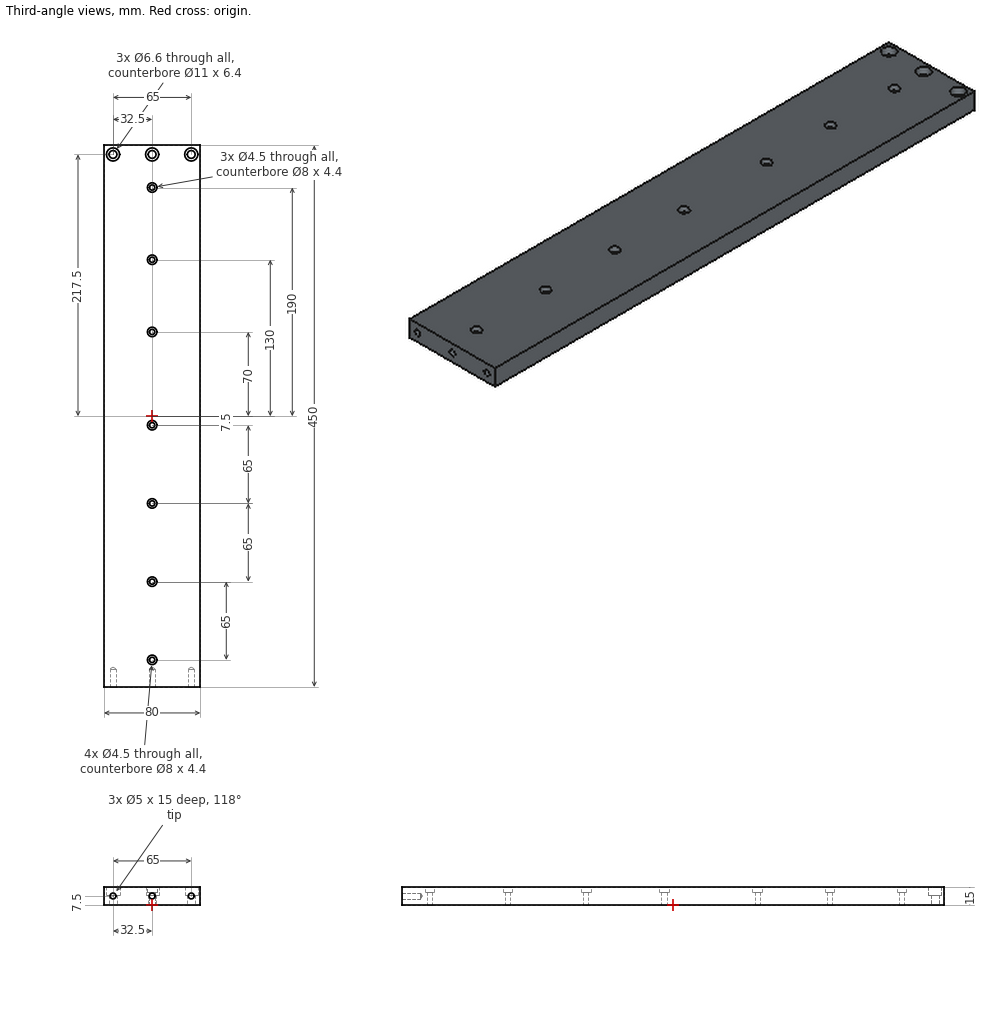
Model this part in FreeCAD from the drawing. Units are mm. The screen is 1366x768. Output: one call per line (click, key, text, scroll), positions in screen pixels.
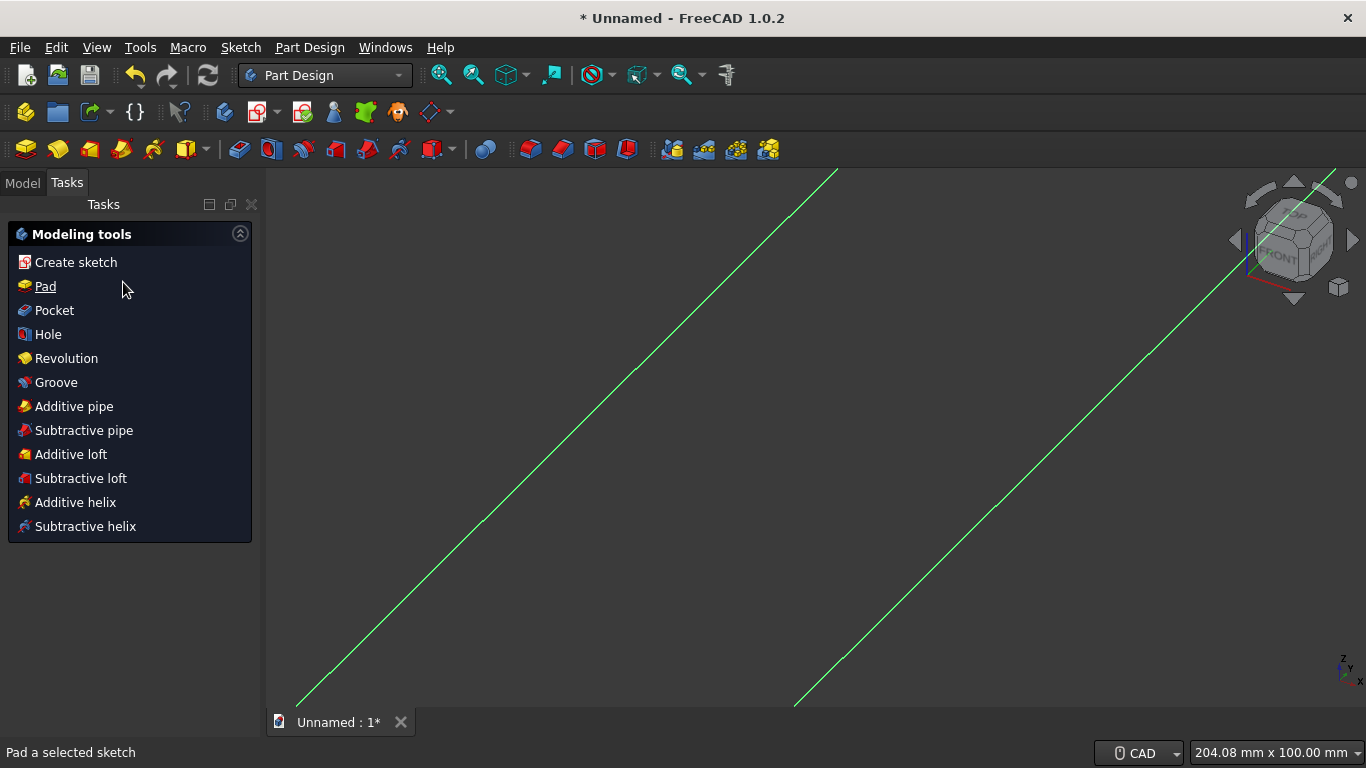
click(26, 150)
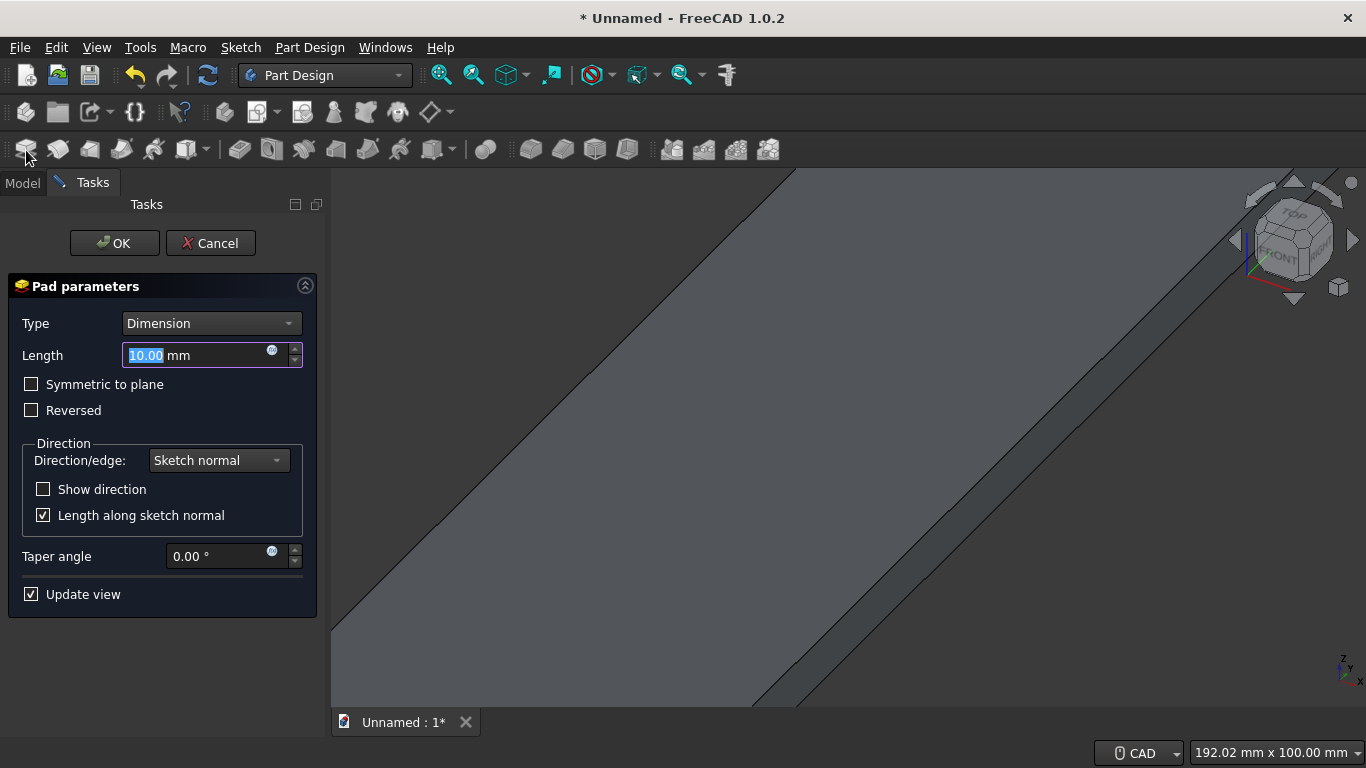
text(15)
key(Tab)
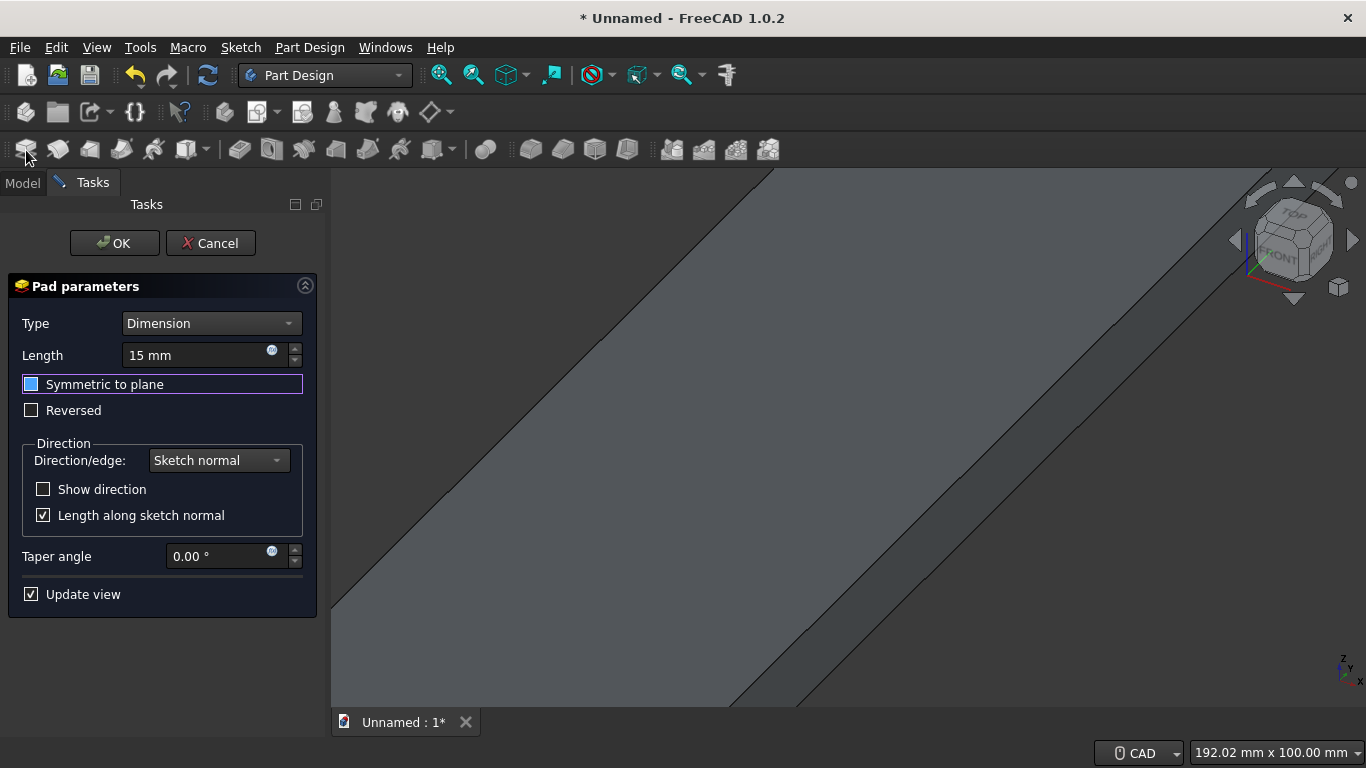
click(115, 243)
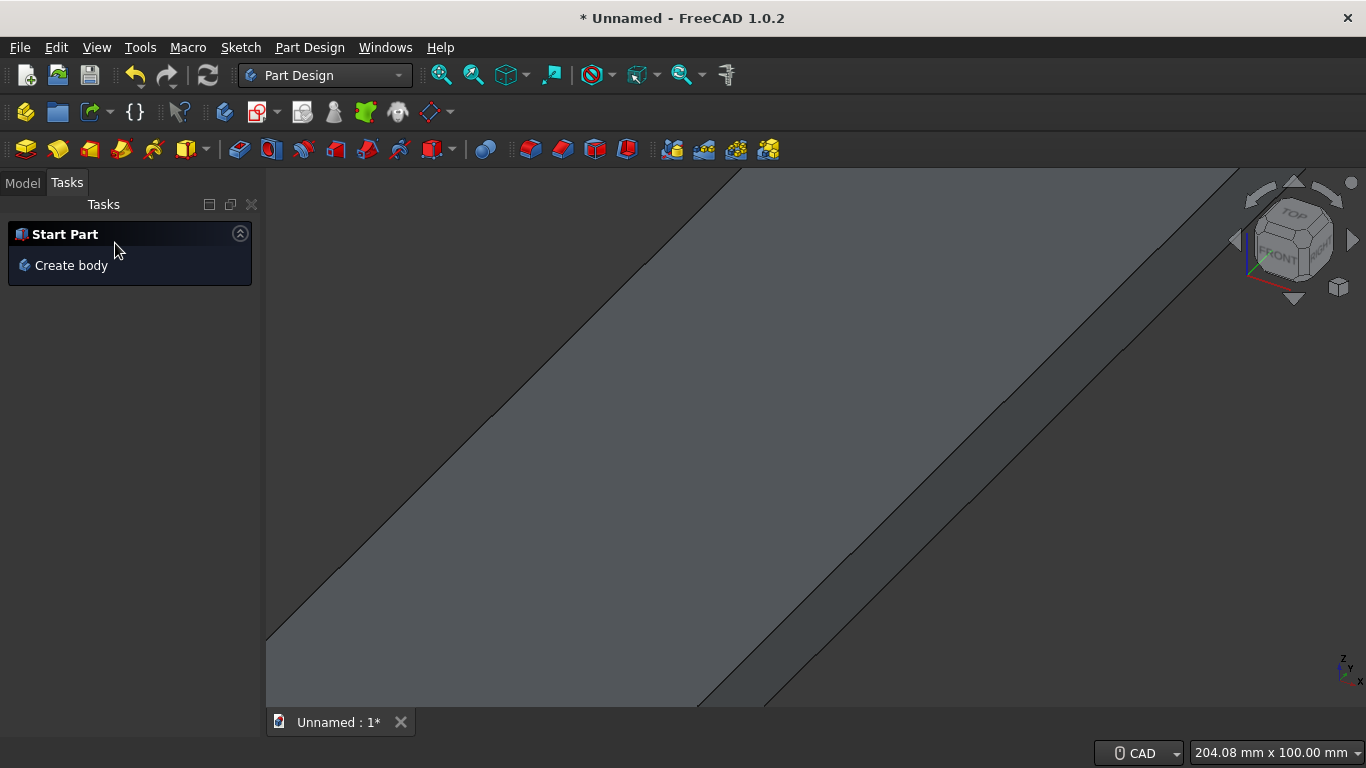
click(442, 76)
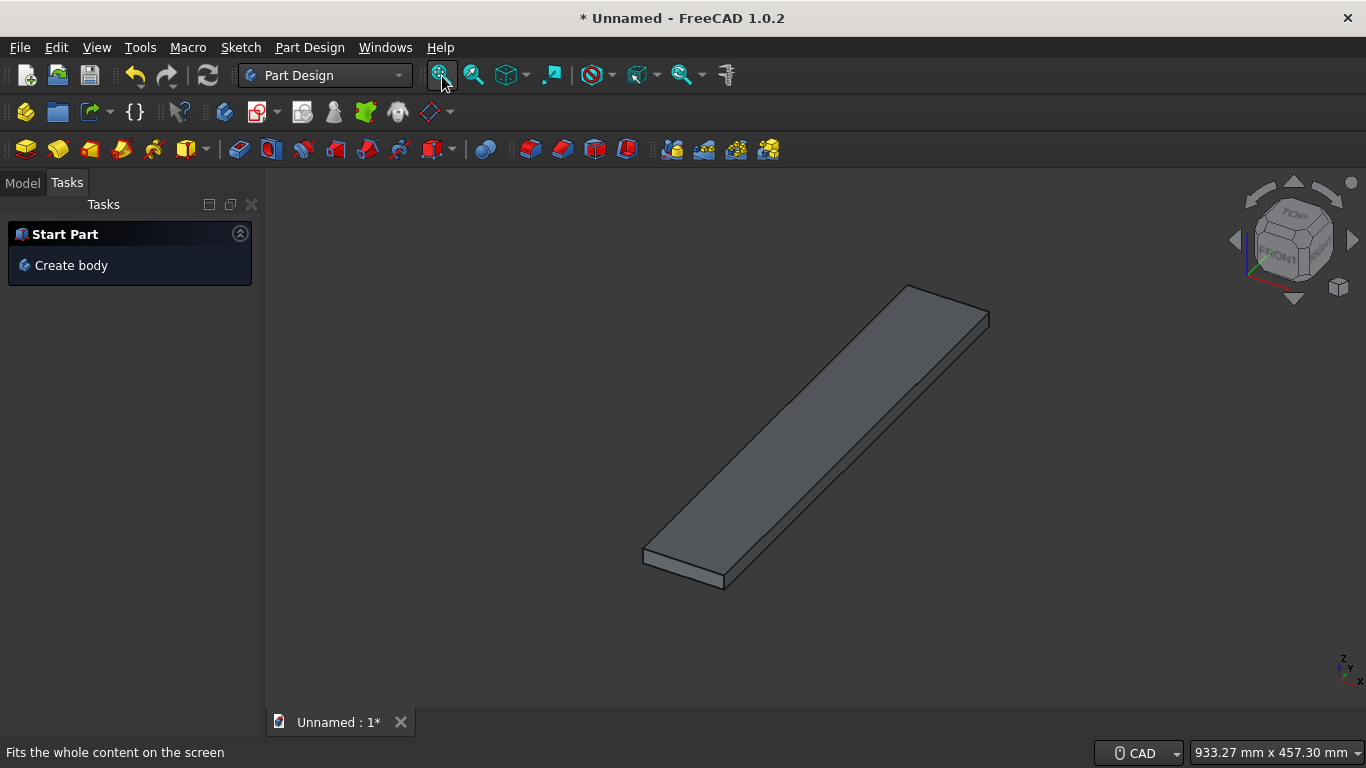
click(892, 354)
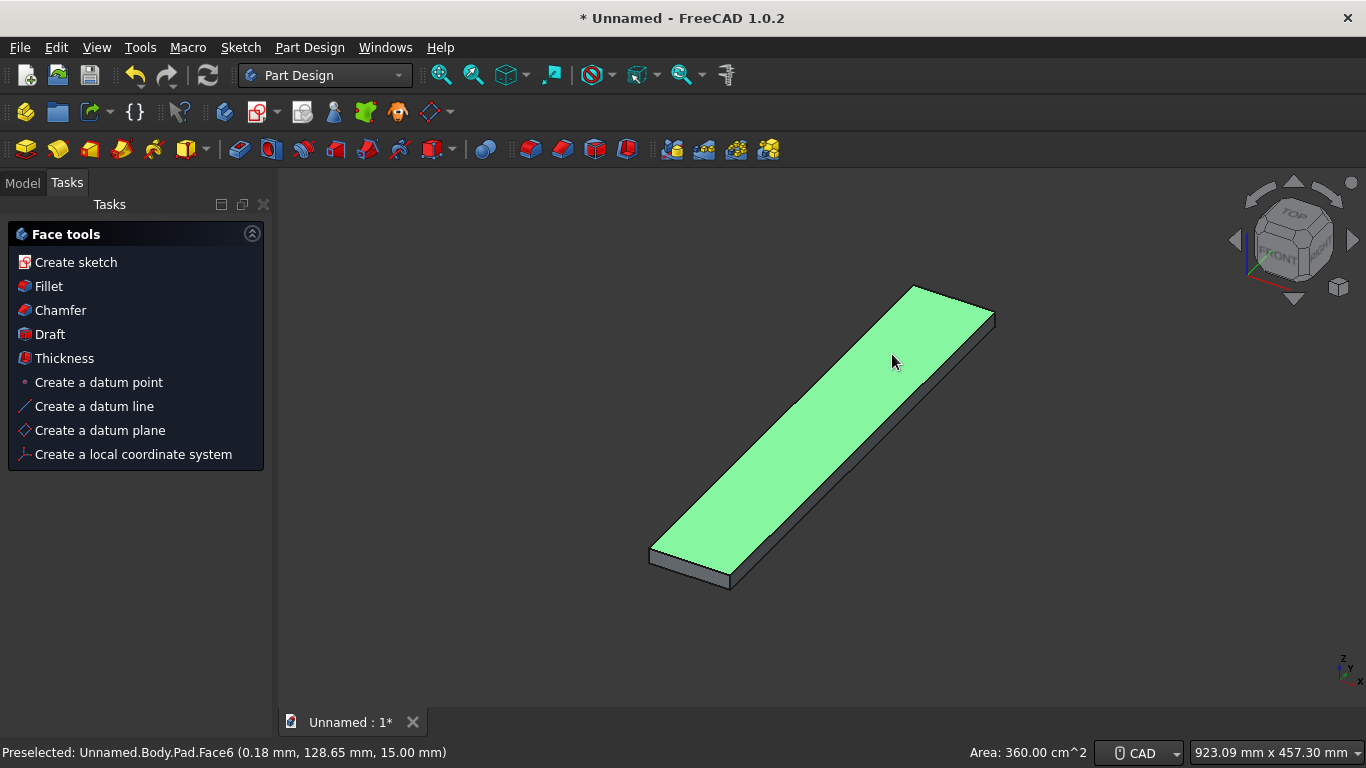
click(258, 112)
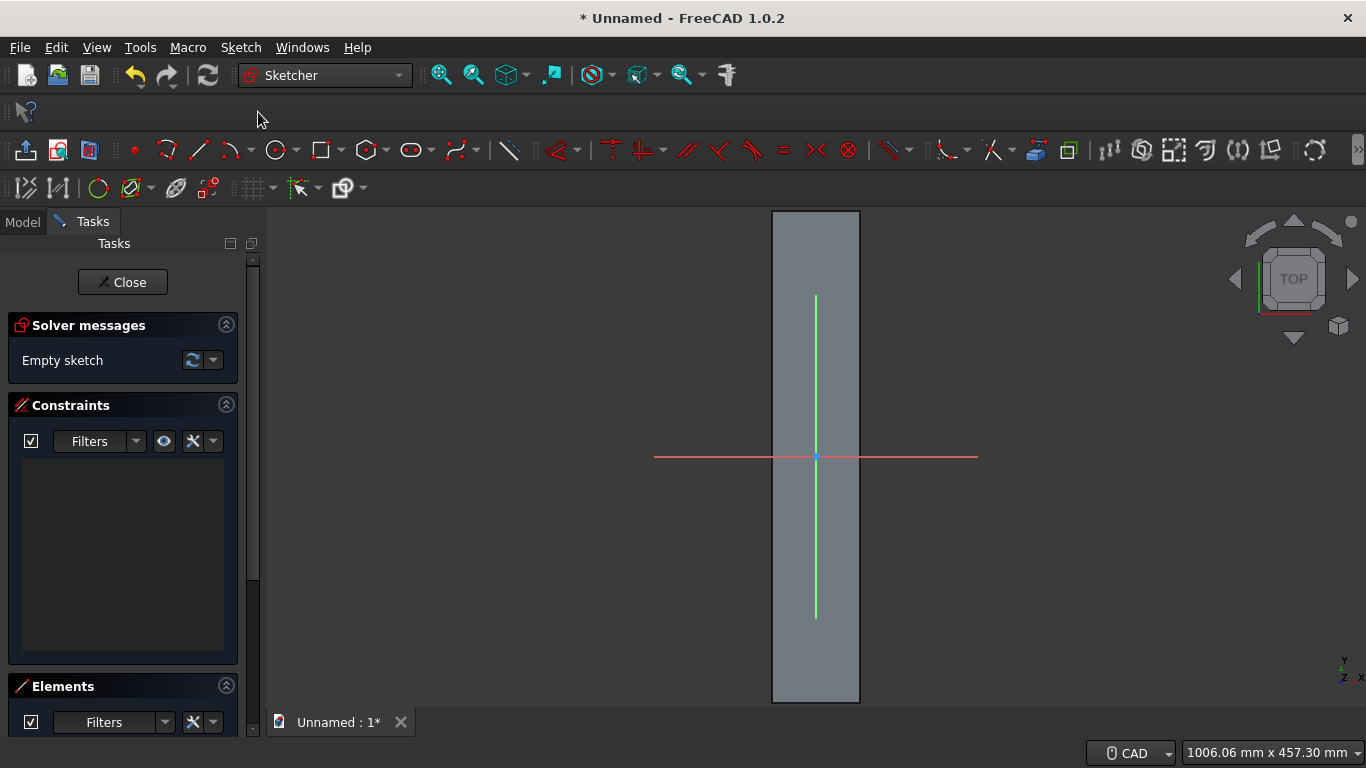
scroll(748, 457, down, 5)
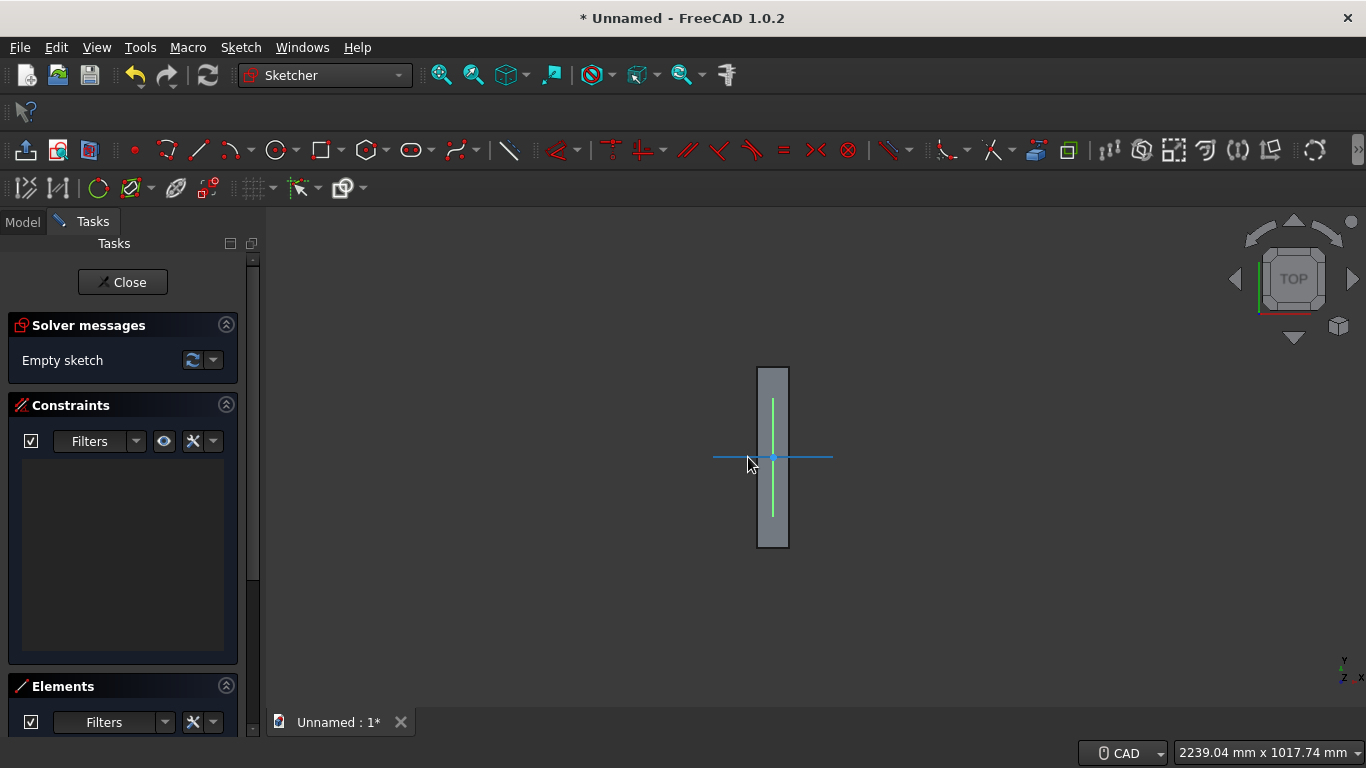
scroll(775, 365, up, 15)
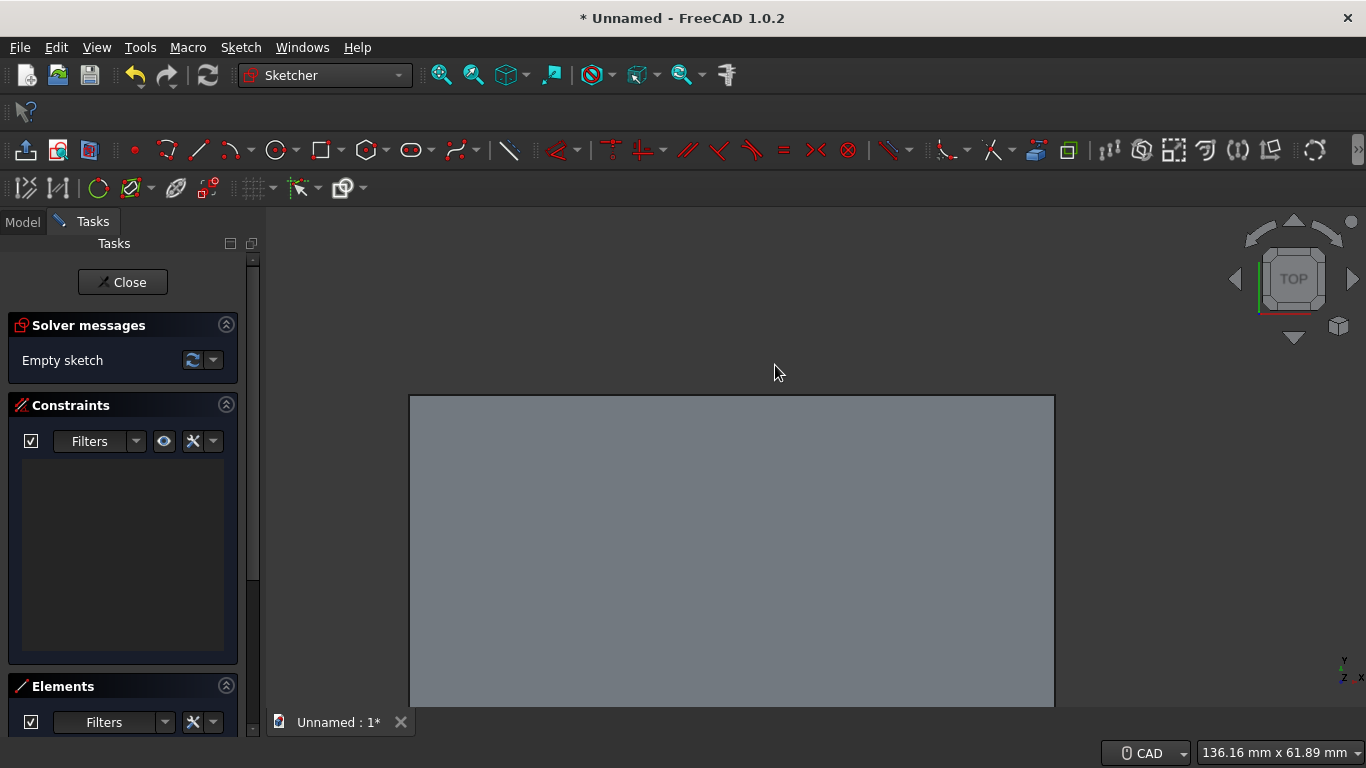
click(276, 150)